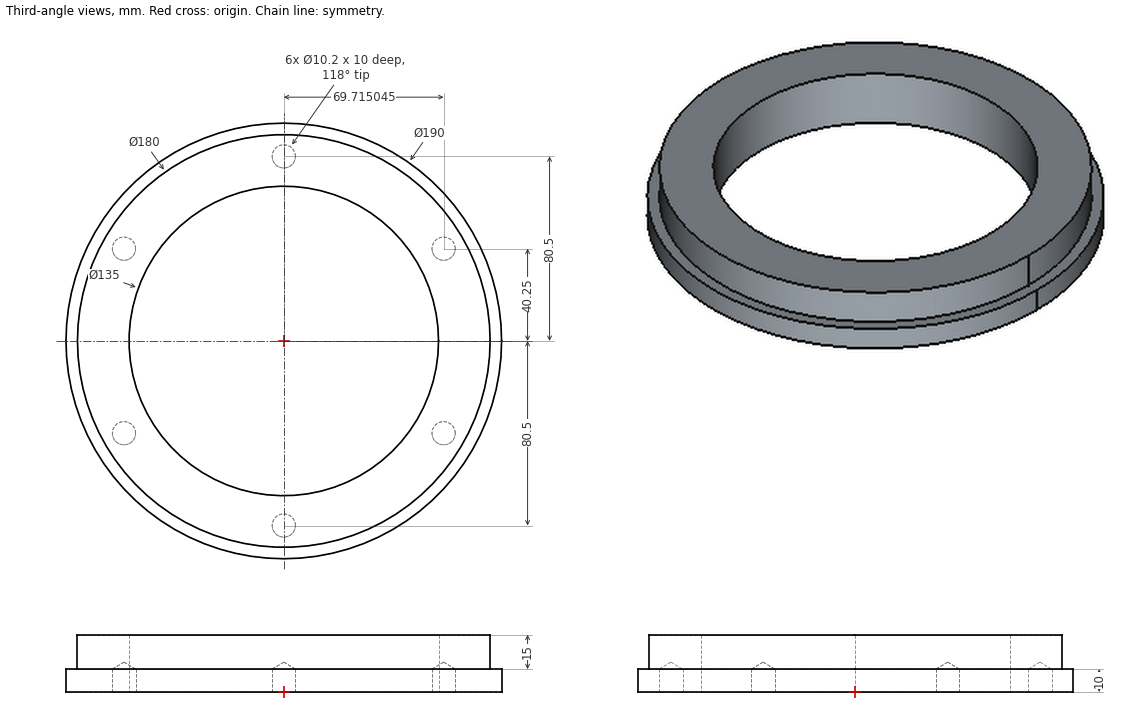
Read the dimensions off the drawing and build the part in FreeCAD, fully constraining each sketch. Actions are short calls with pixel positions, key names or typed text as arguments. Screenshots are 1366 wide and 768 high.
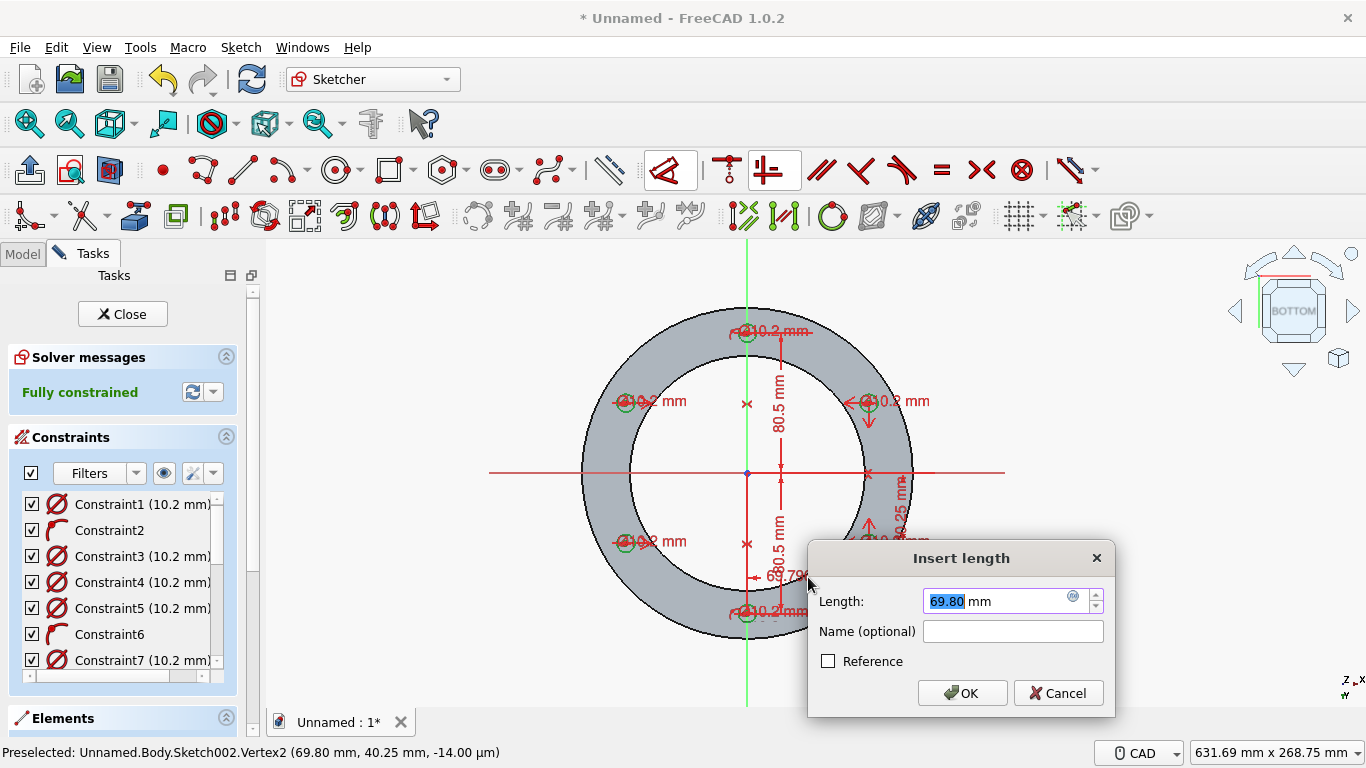
text(69.715045)
key(Return)
key(Escape)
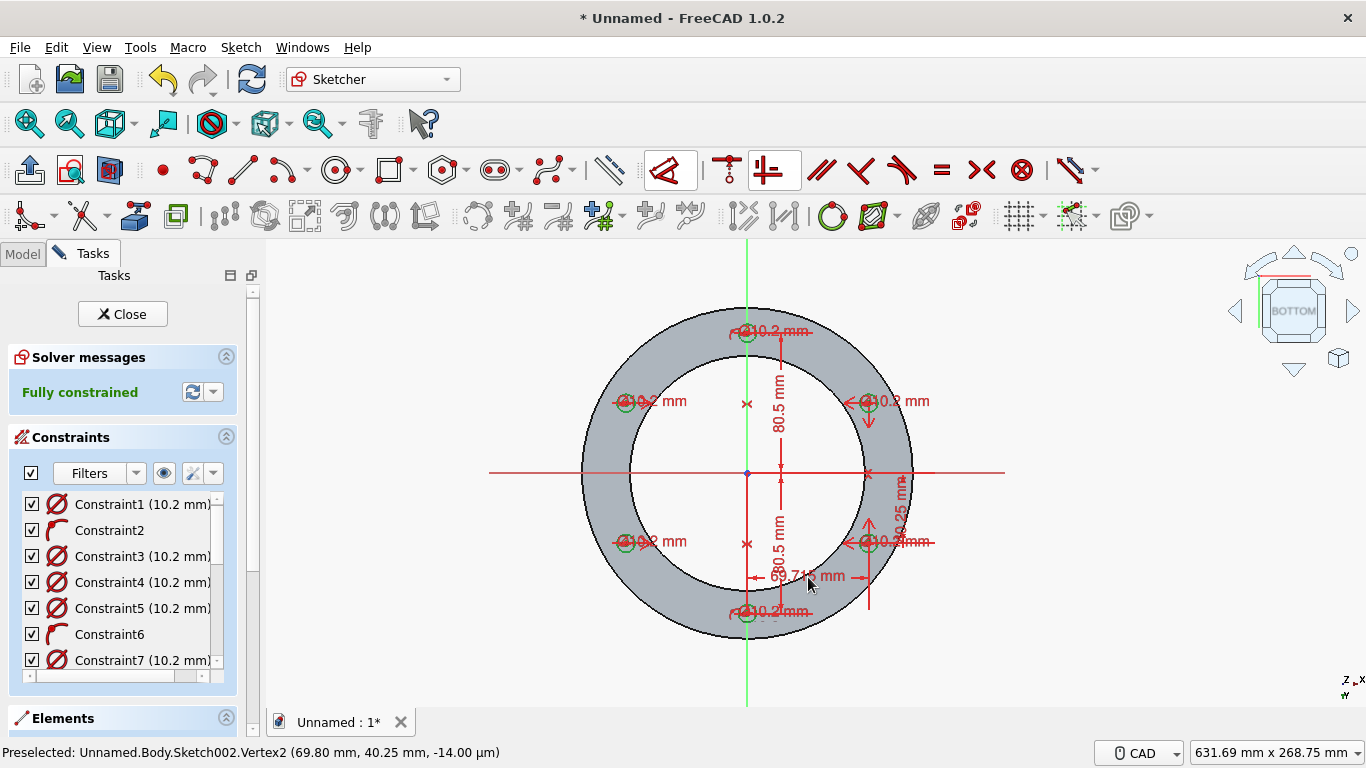
click(123, 314)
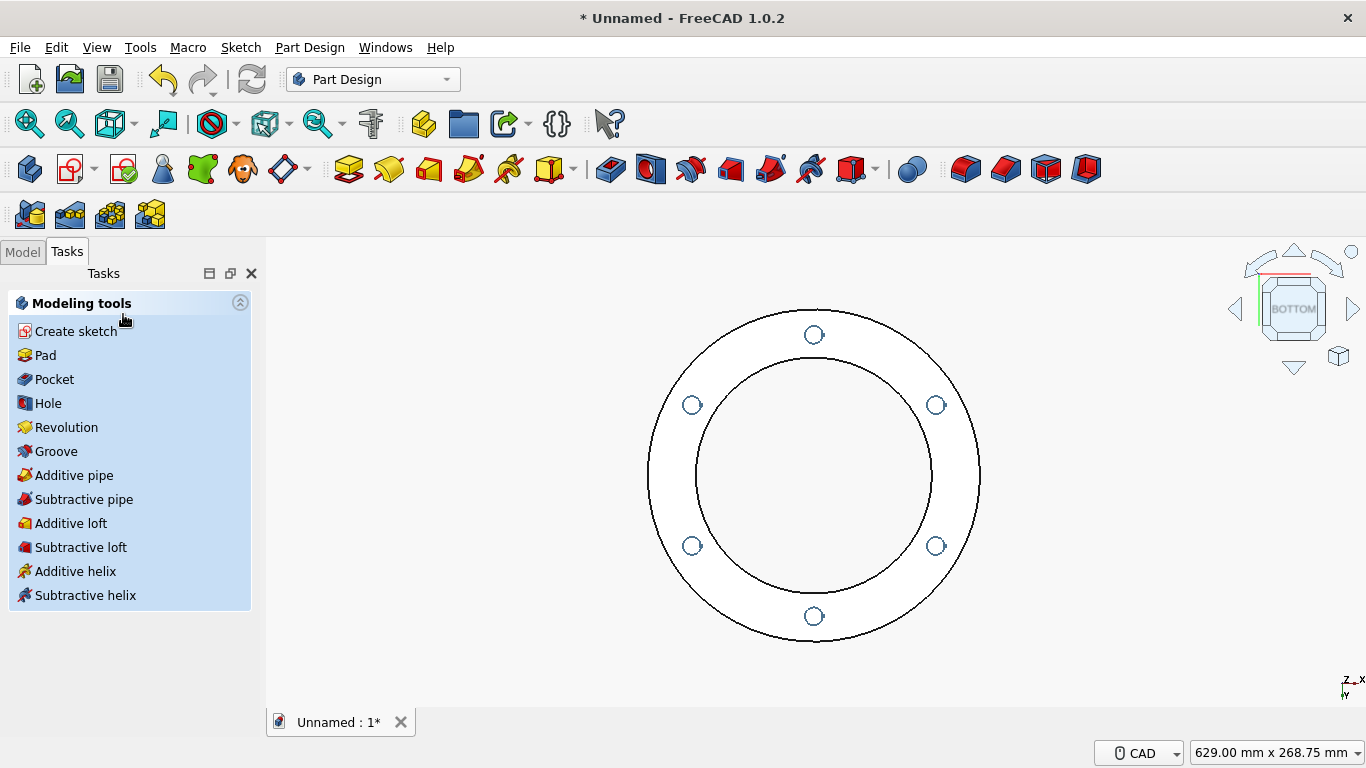
click(652, 170)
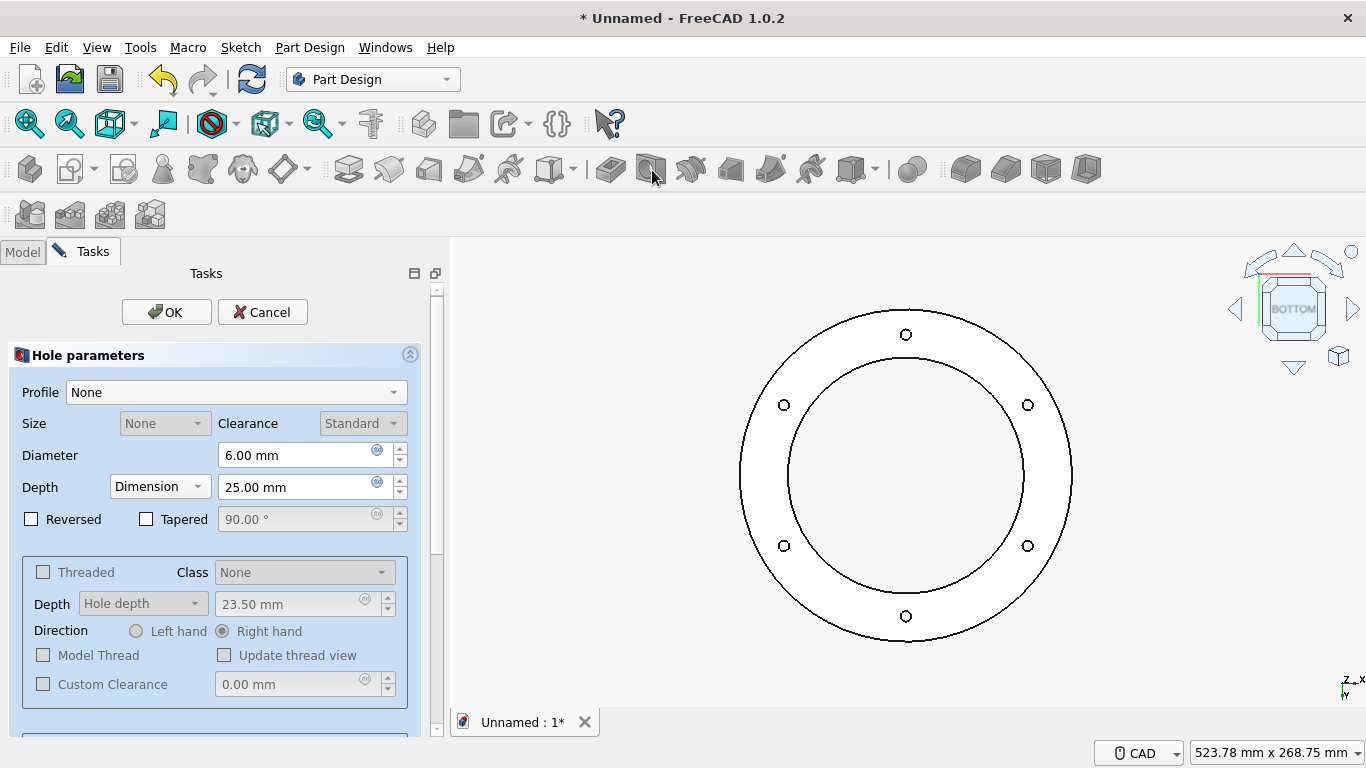
triple_click(305, 455)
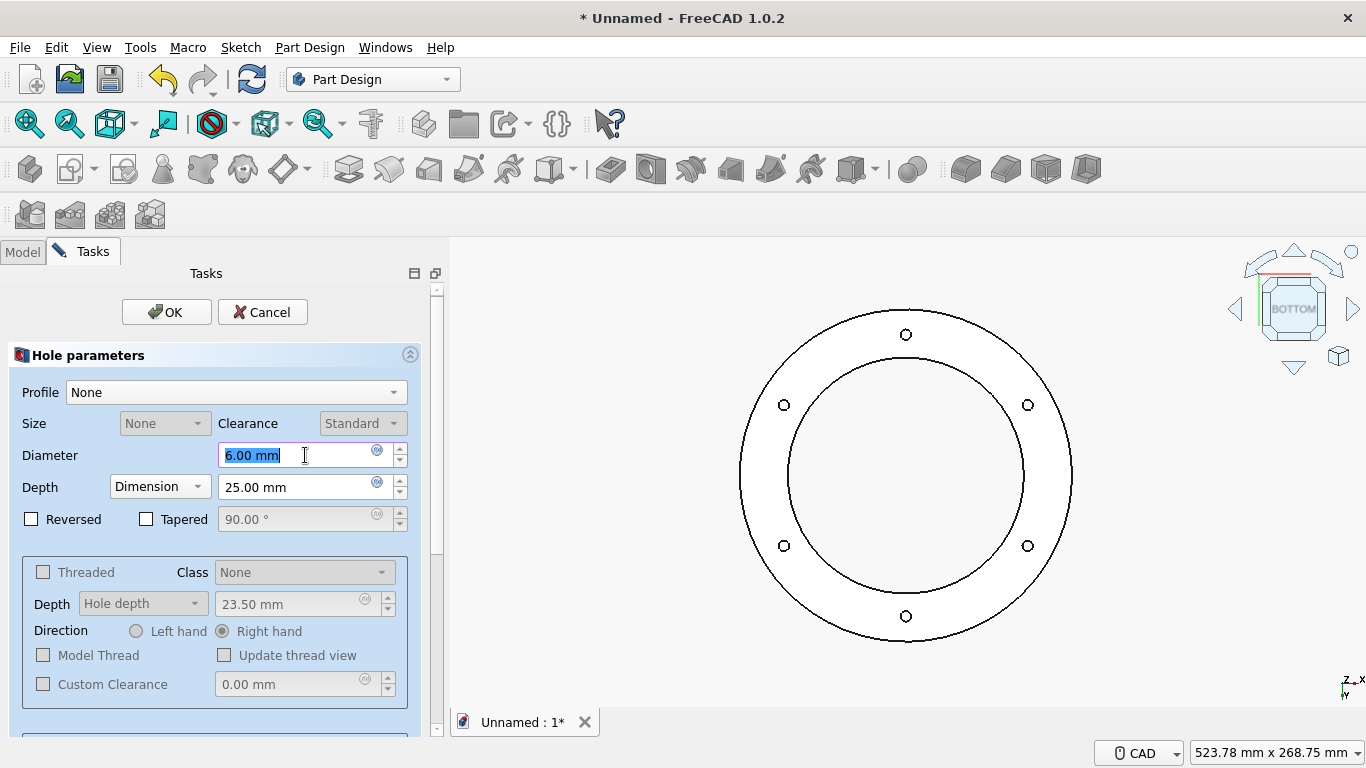
text(10.2)
key(Tab)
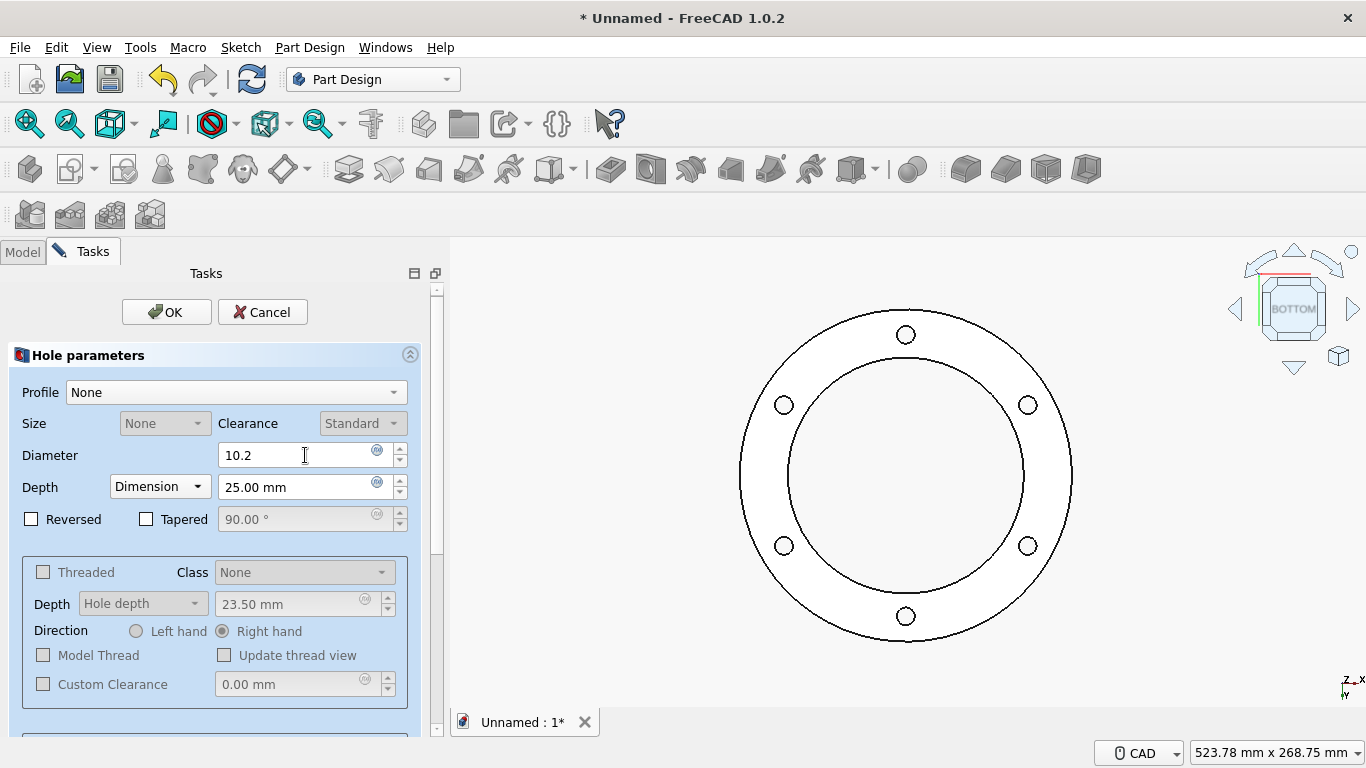
triple_click(305, 487)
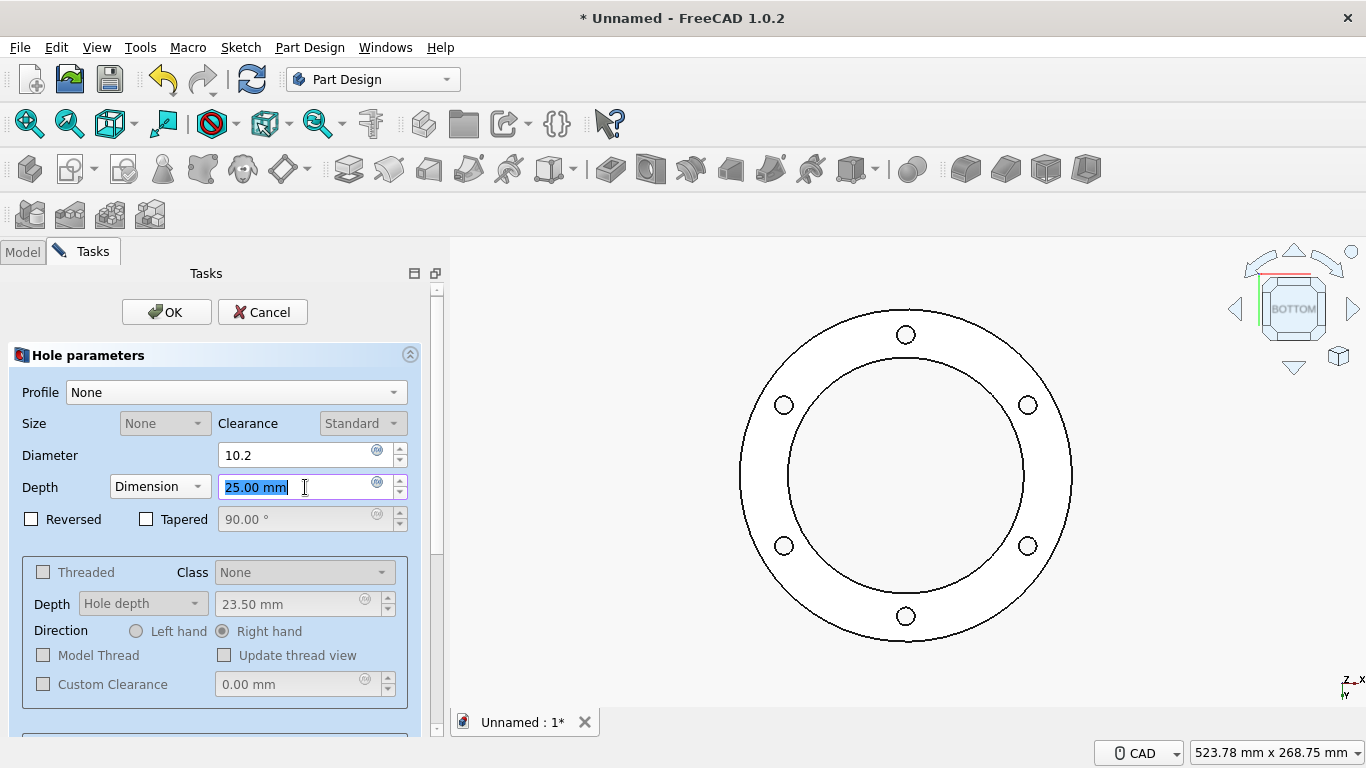
text(10)
key(Tab)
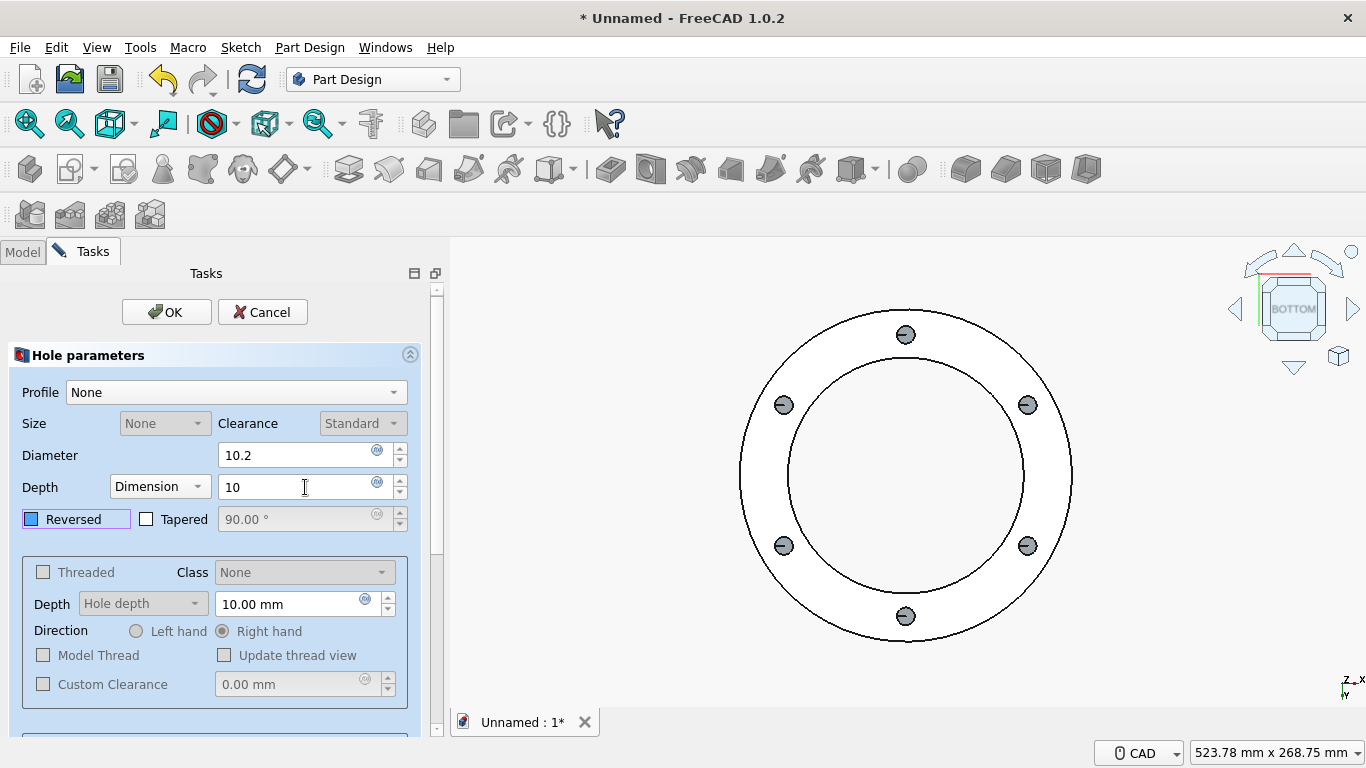
click(167, 312)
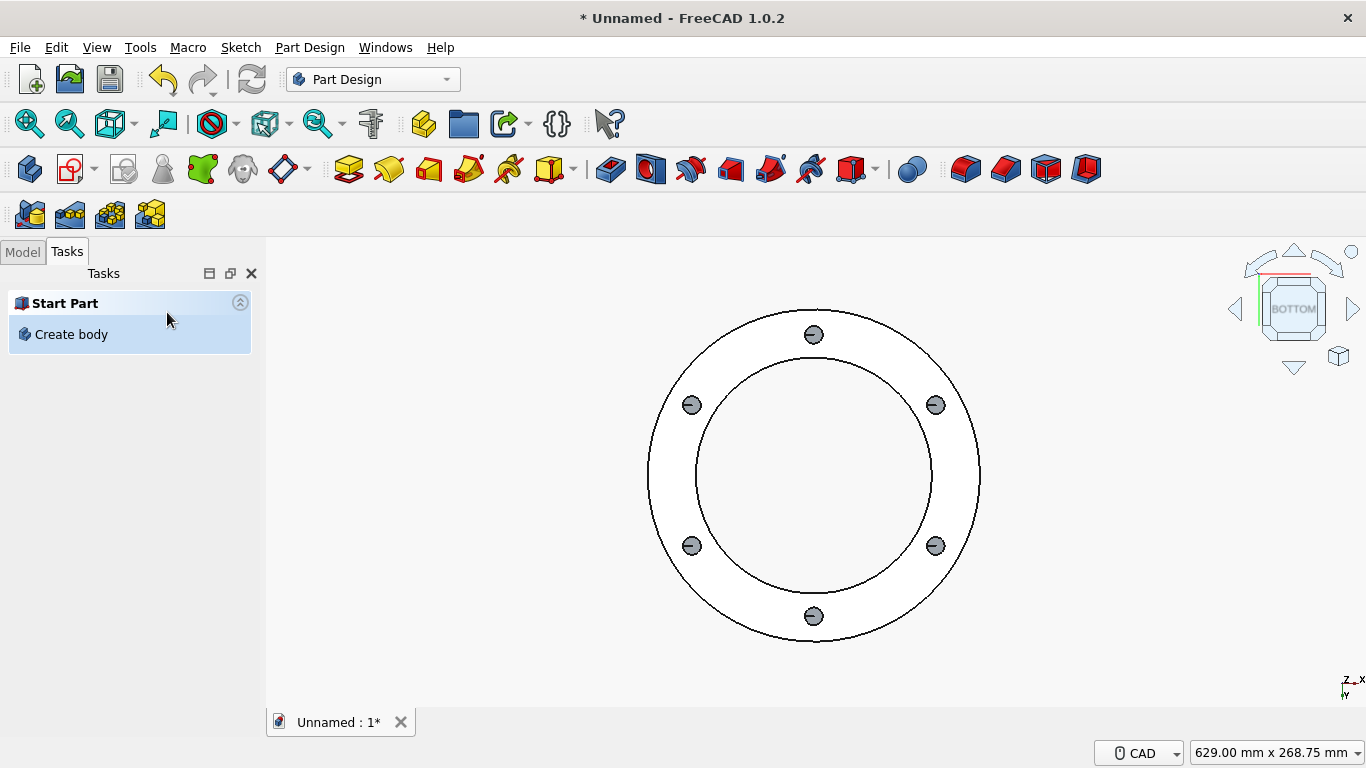
key(0)